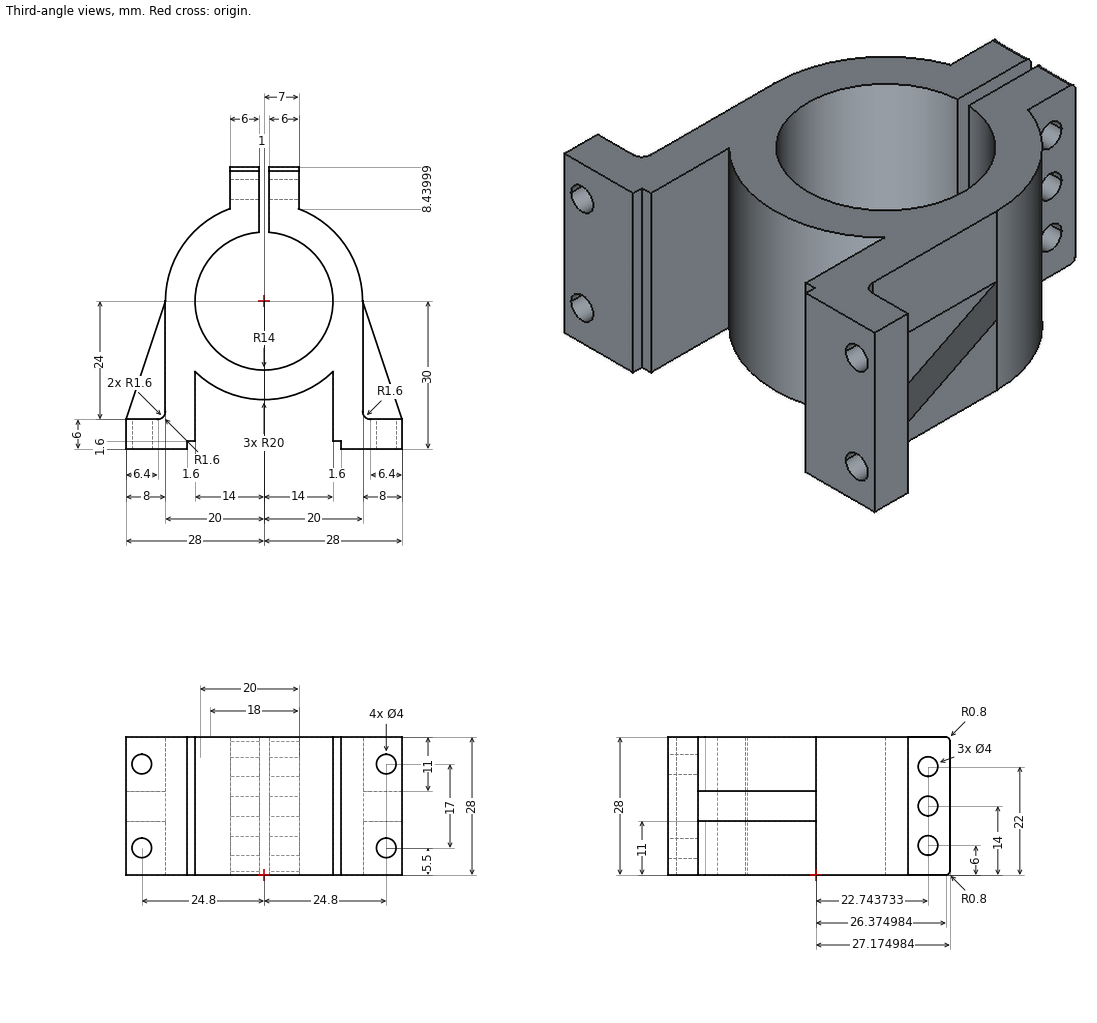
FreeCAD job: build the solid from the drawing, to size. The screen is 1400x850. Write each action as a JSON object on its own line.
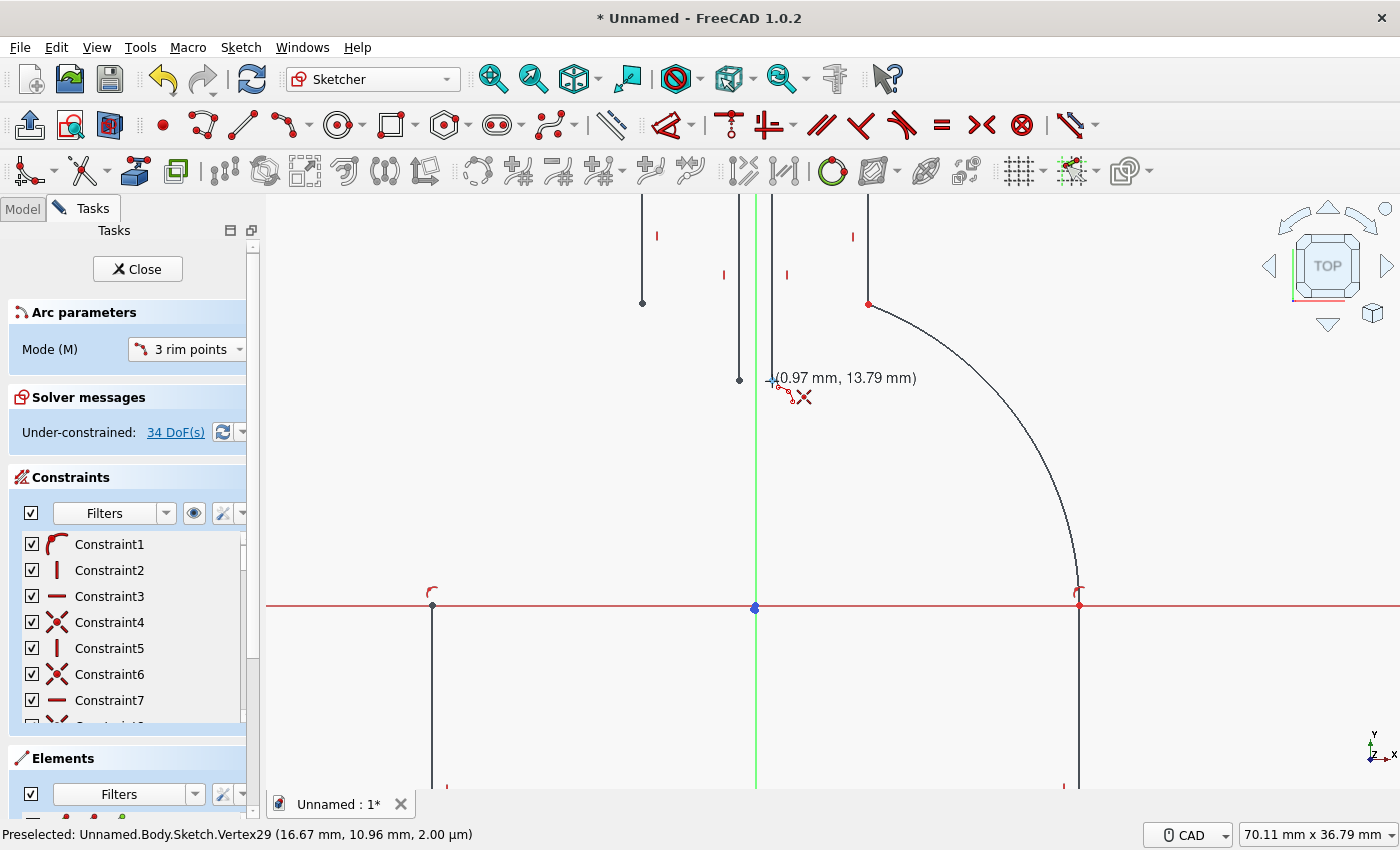
{"action": "left_click", "coordinate": [772, 381]}
{"action": "left_click", "coordinate": [739, 381]}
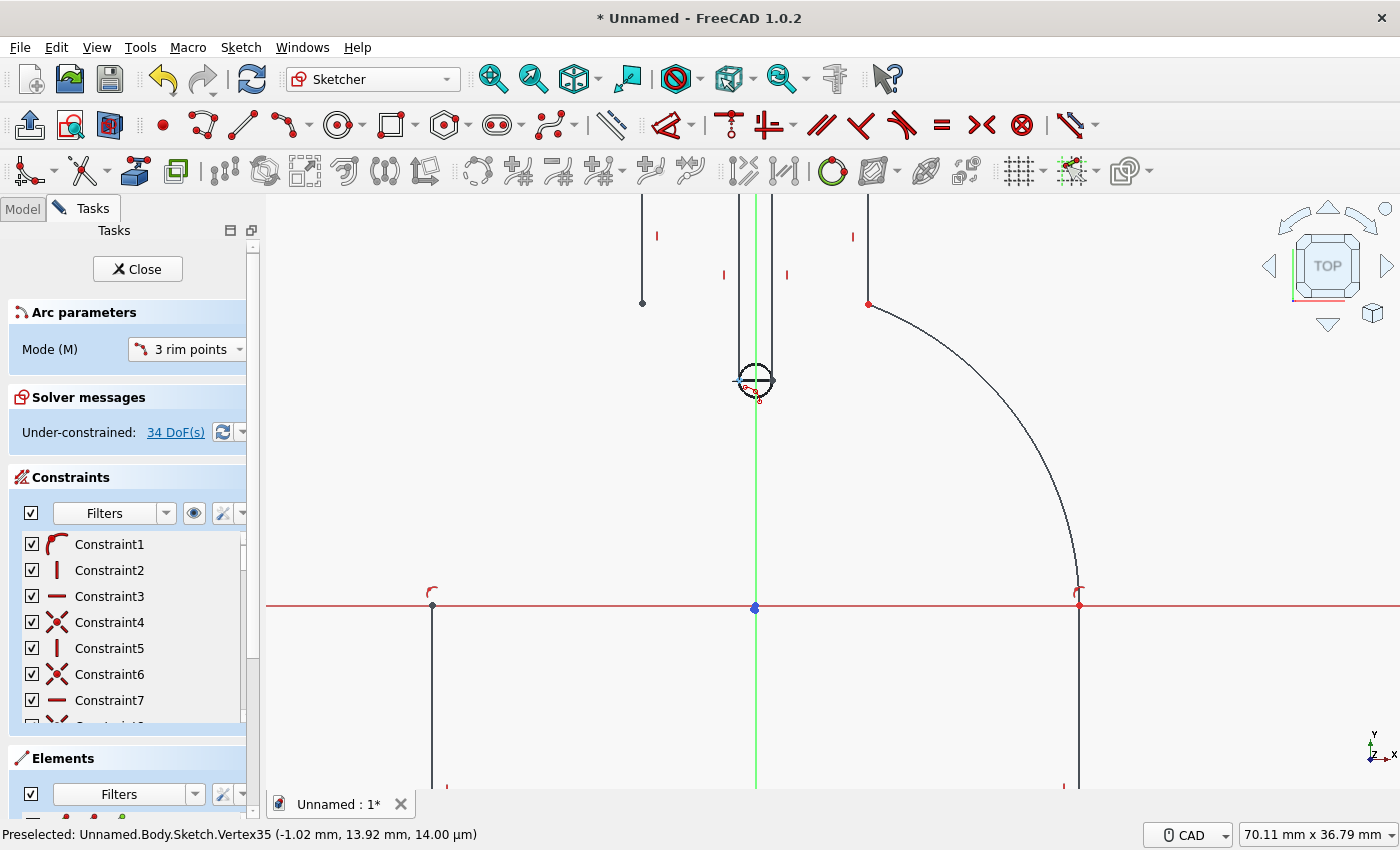
{"action": "scroll", "coordinate": [772, 380], "scroll_direction": "down", "scroll_amount": 4}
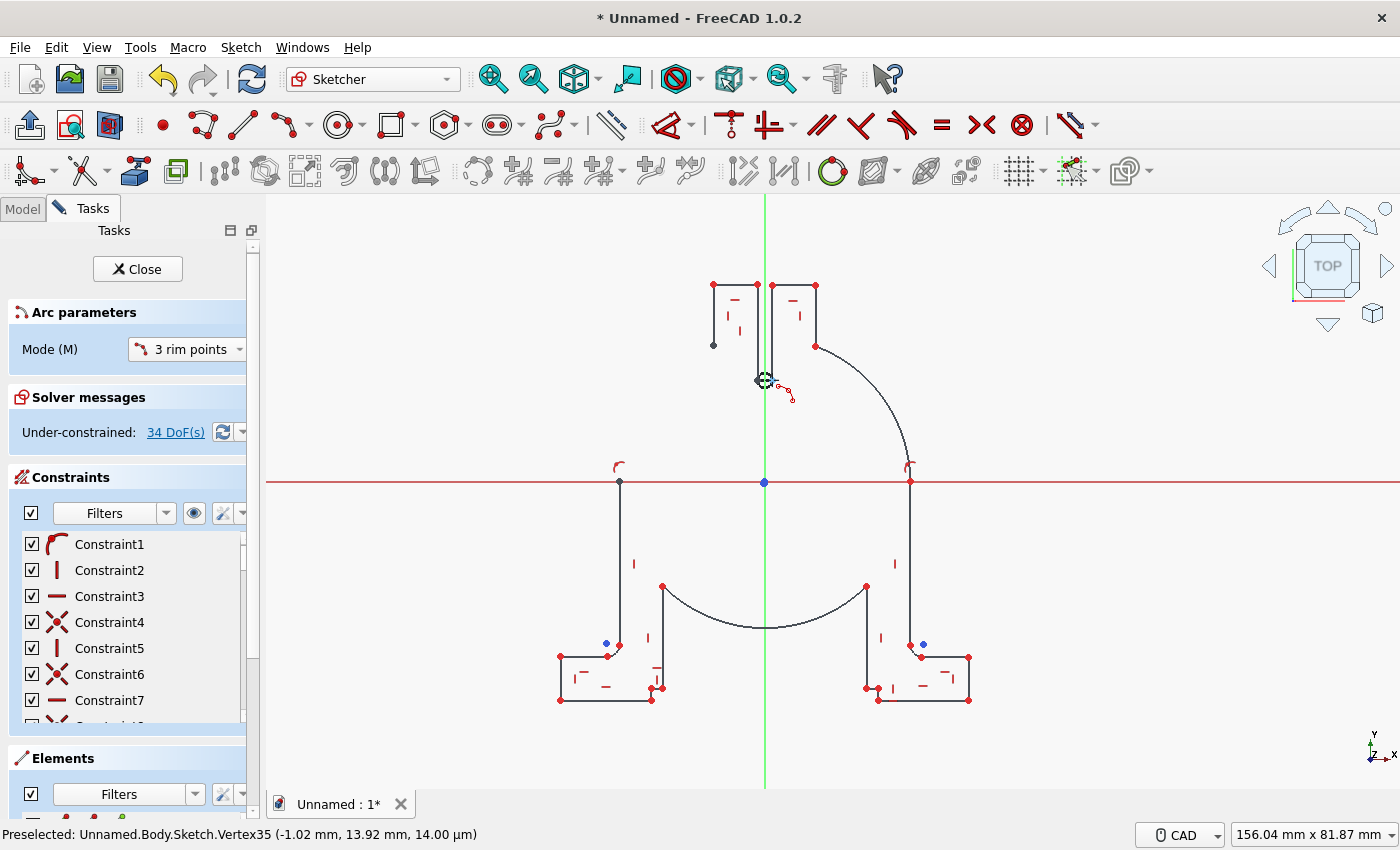
{"action": "left_click", "coordinate": [706, 565]}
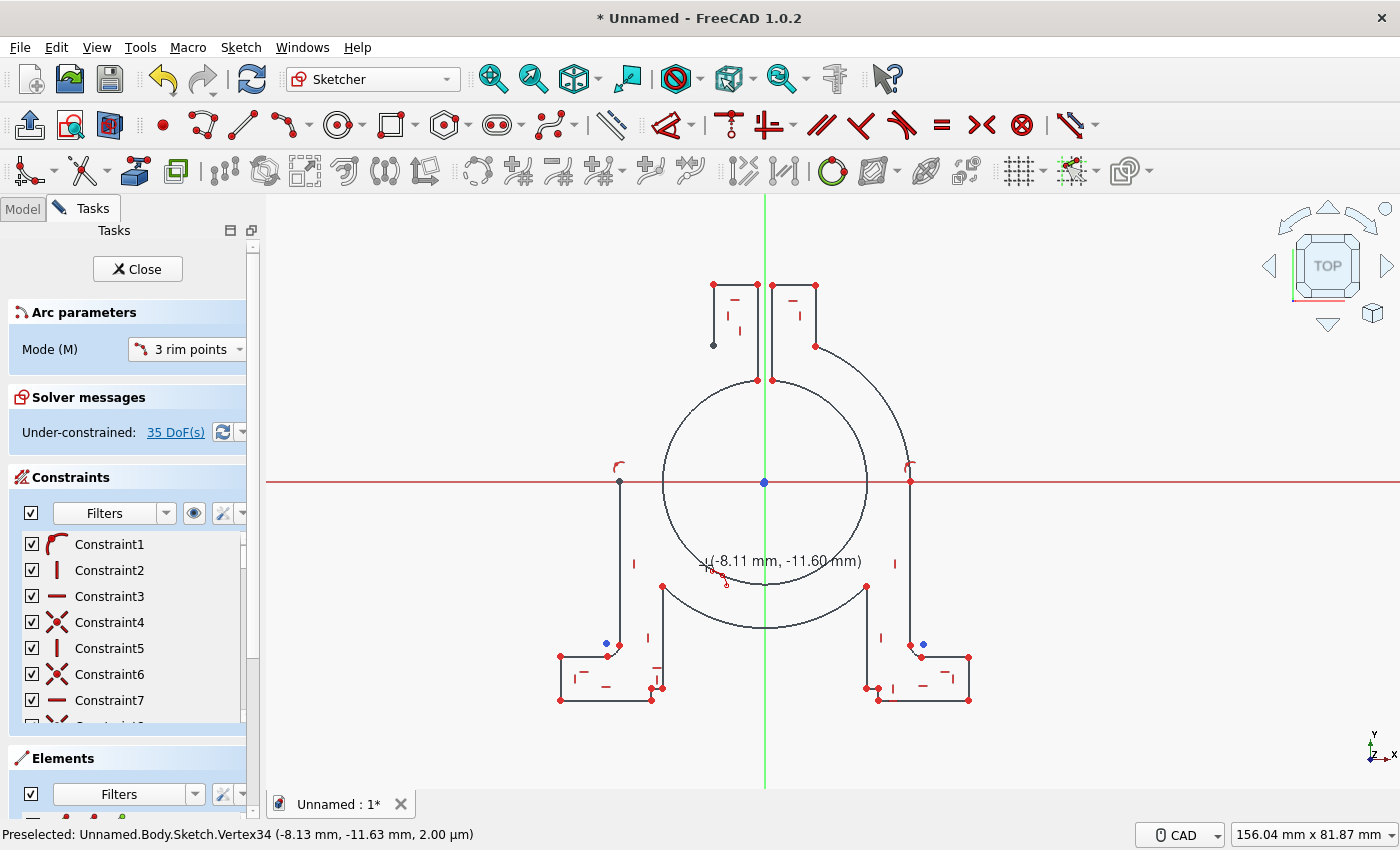
{"action": "left_click", "coordinate": [714, 346]}
{"action": "left_click", "coordinate": [620, 482]}
{"action": "left_click", "coordinate": [646, 399]}
{"action": "key", "text": "Escape"}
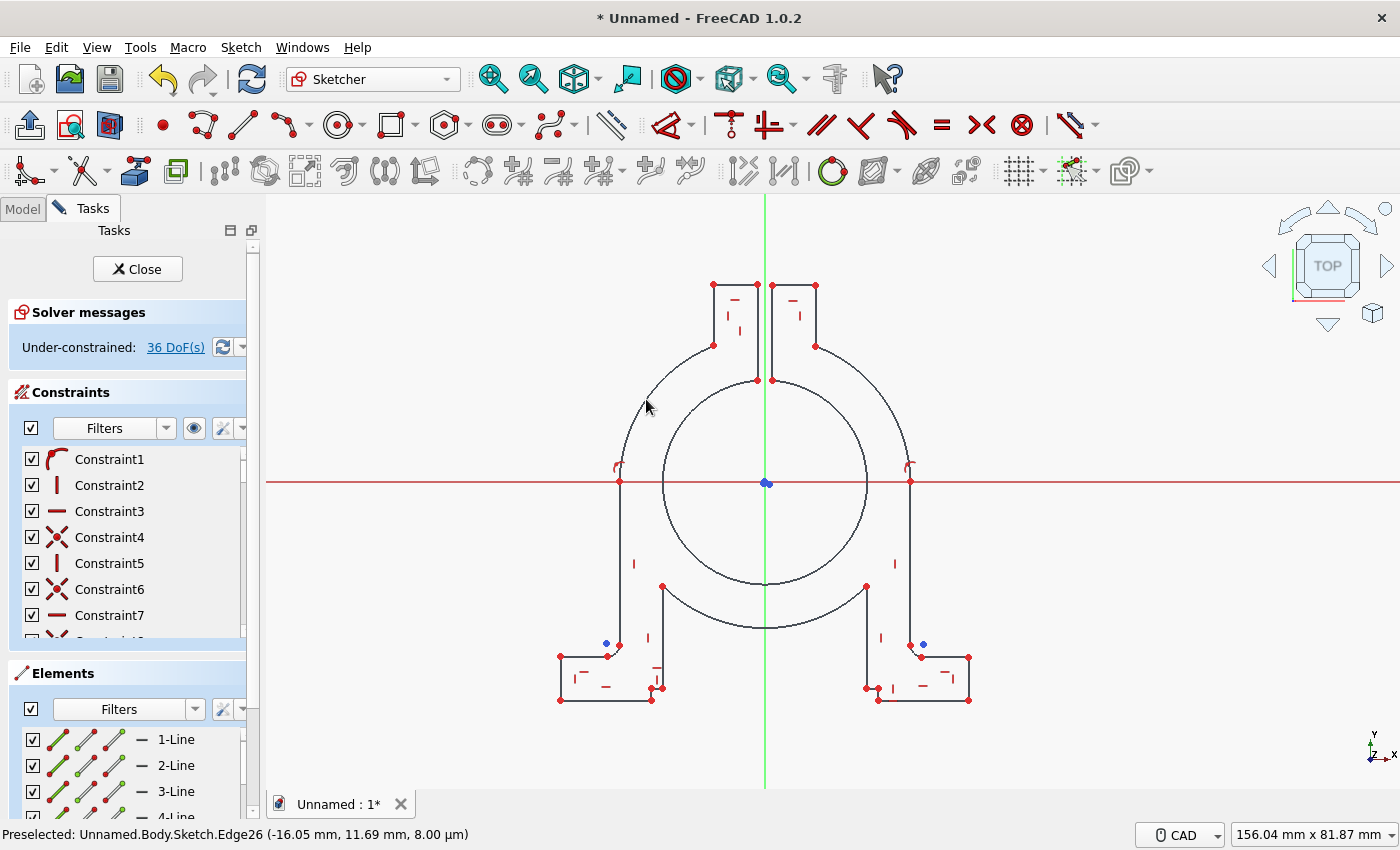
{"action": "left_click", "coordinate": [620, 531]}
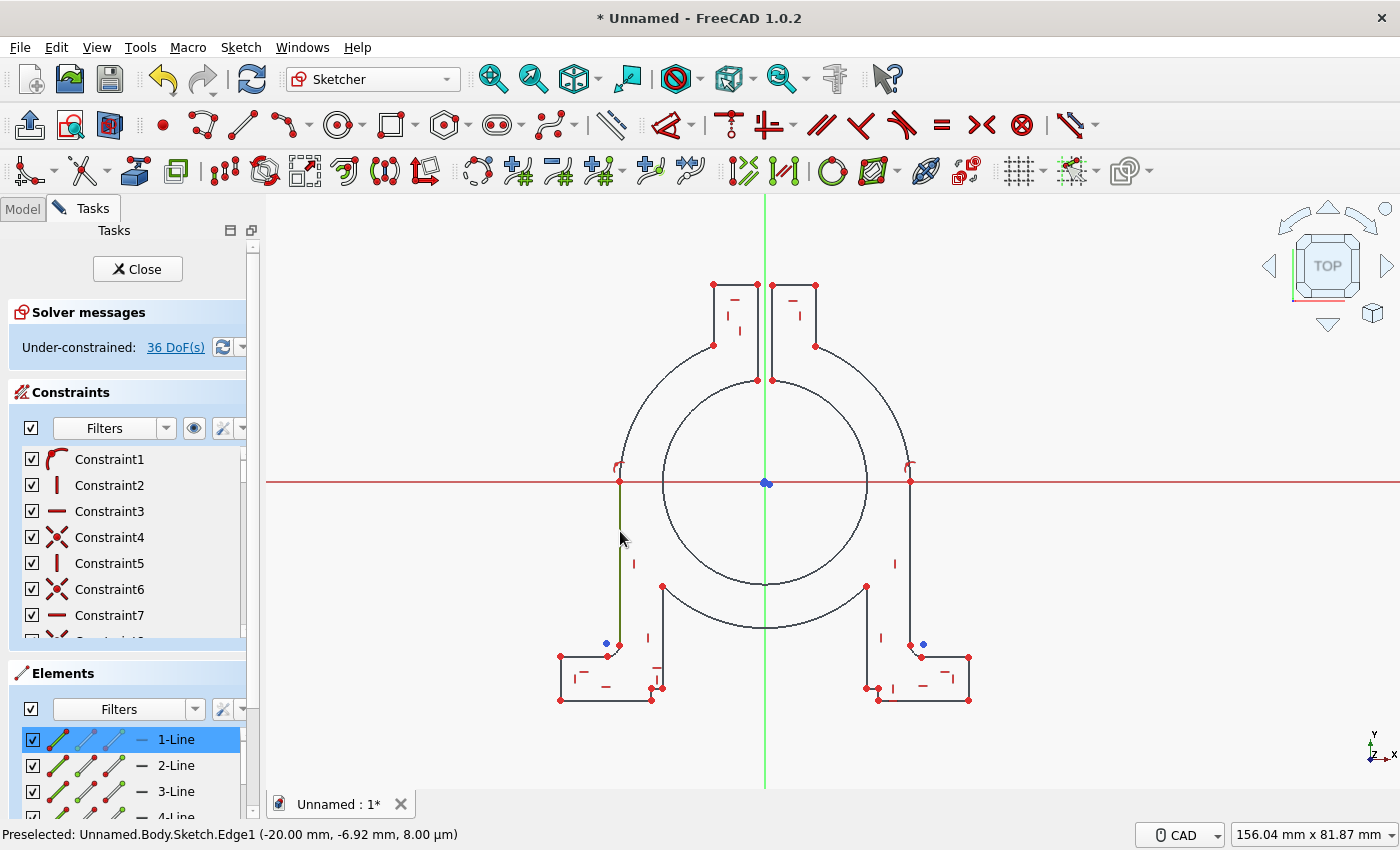
{"action": "scroll", "coordinate": [615, 654], "scroll_direction": "up", "scroll_amount": 3}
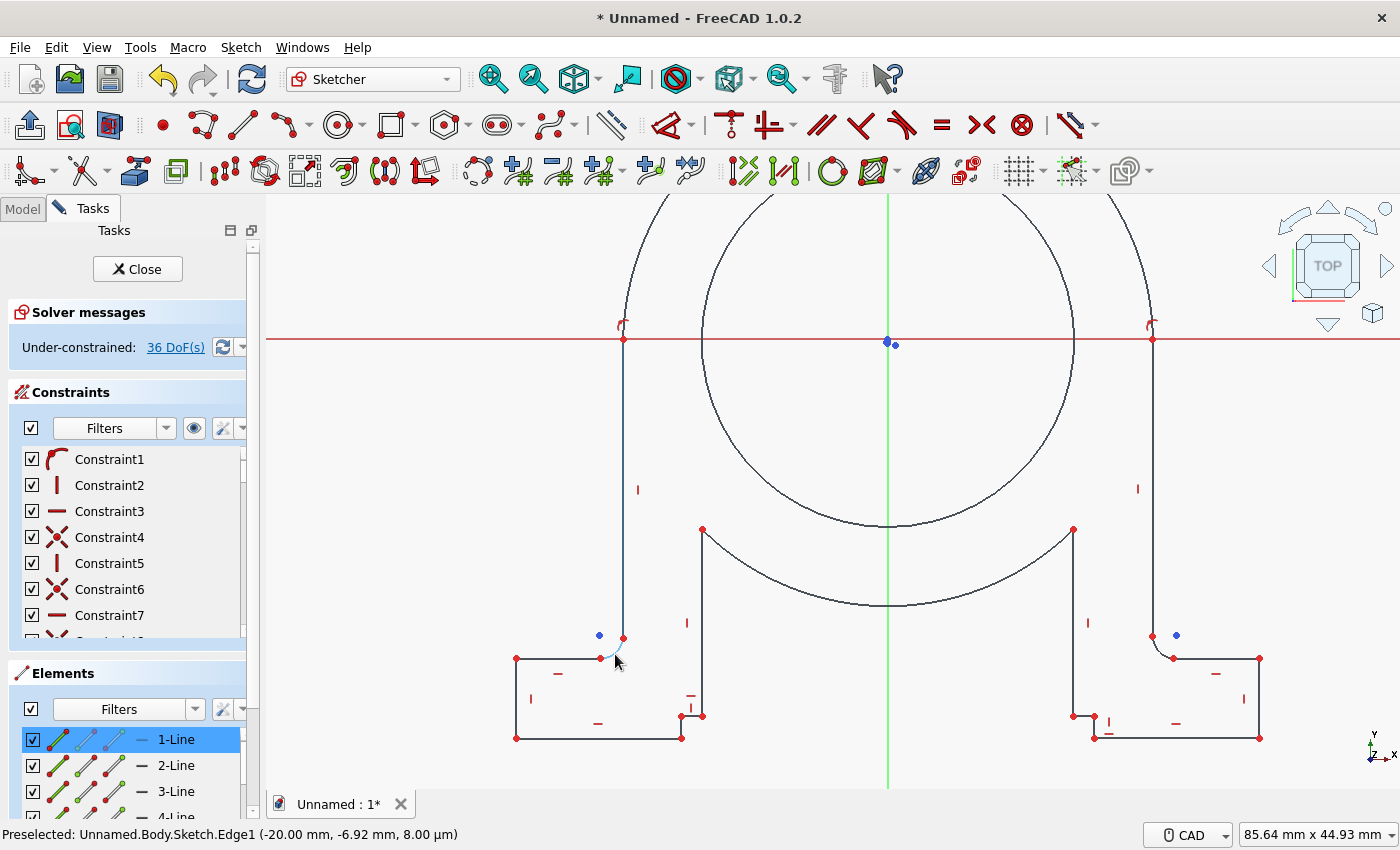
{"action": "left_click", "coordinate": [616, 653]}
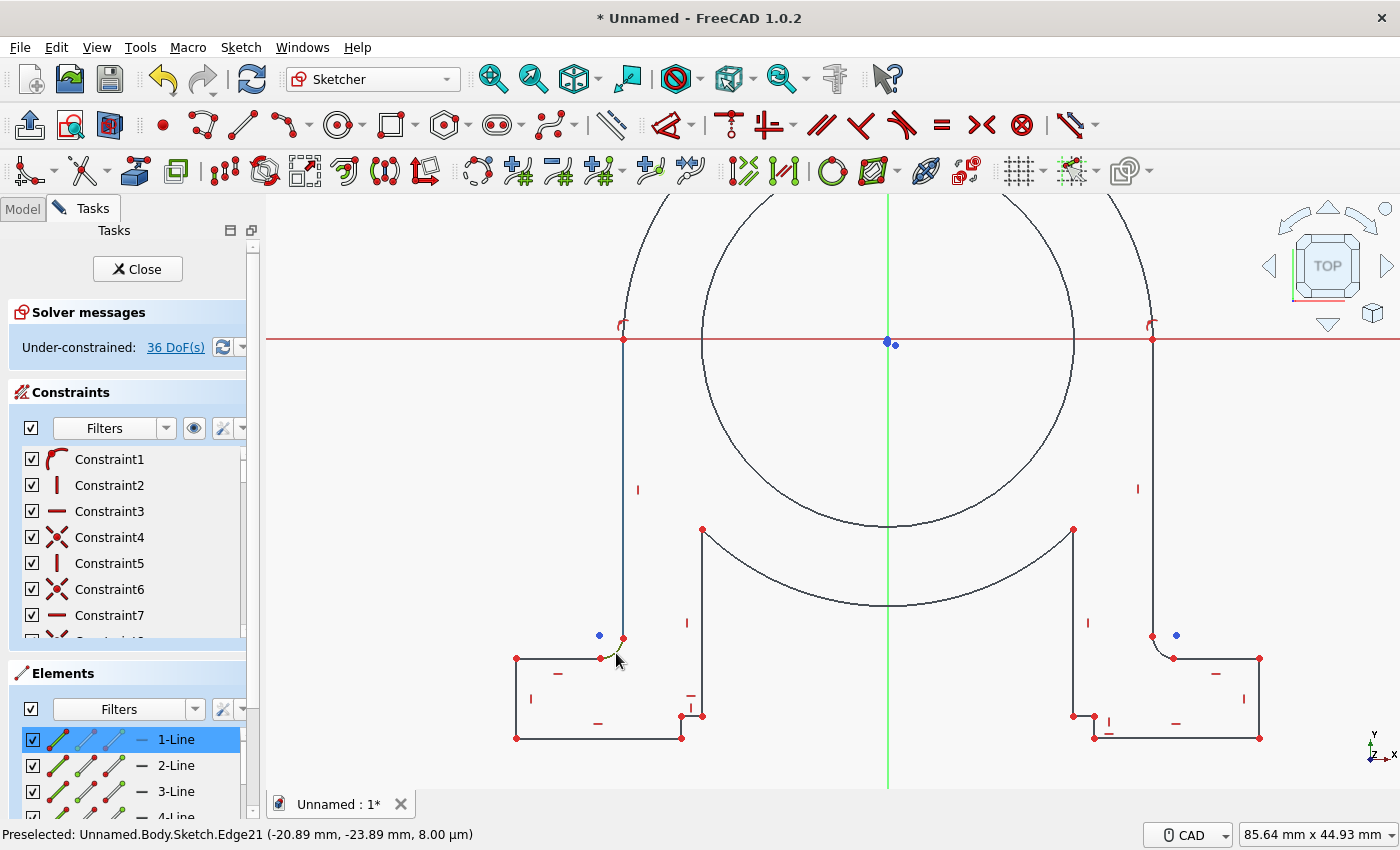
{"action": "left_click", "coordinate": [902, 126]}